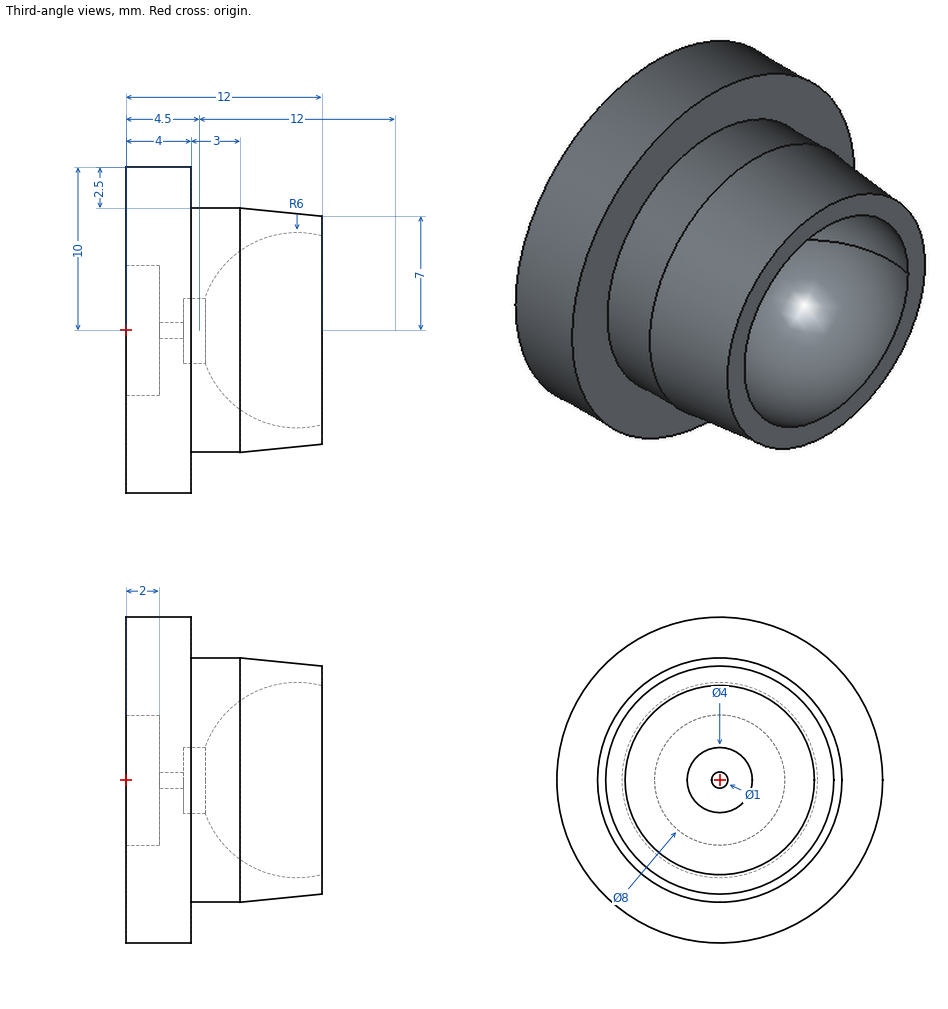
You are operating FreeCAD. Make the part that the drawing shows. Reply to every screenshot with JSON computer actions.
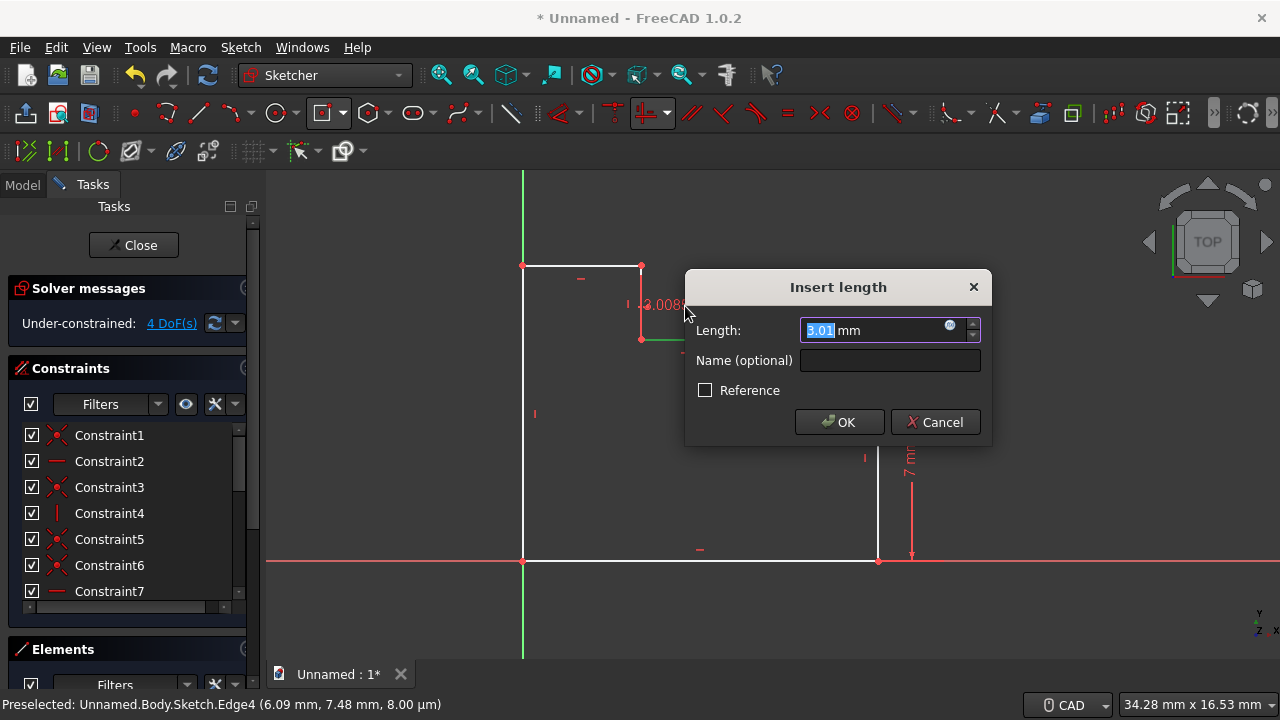
{"action": "type", "text": "3"}
{"action": "key", "text": "Return"}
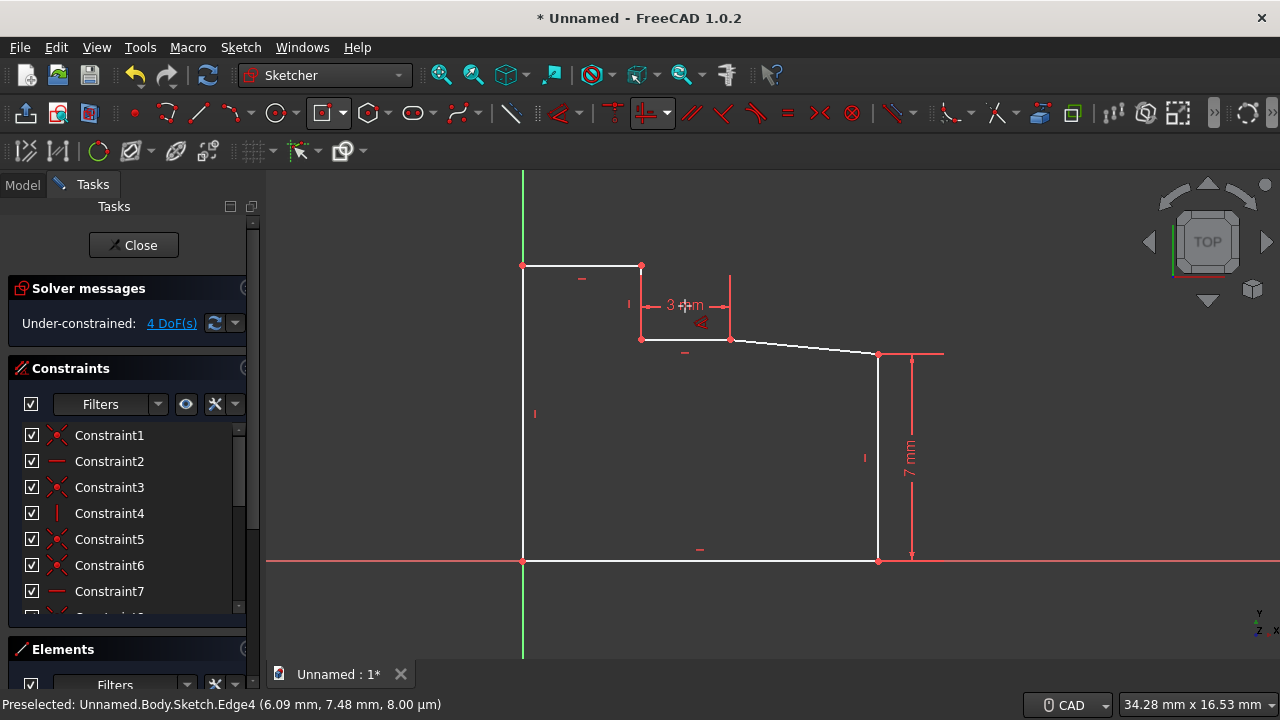
{"action": "left_click", "coordinate": [606, 266]}
{"action": "left_click", "coordinate": [582, 232]}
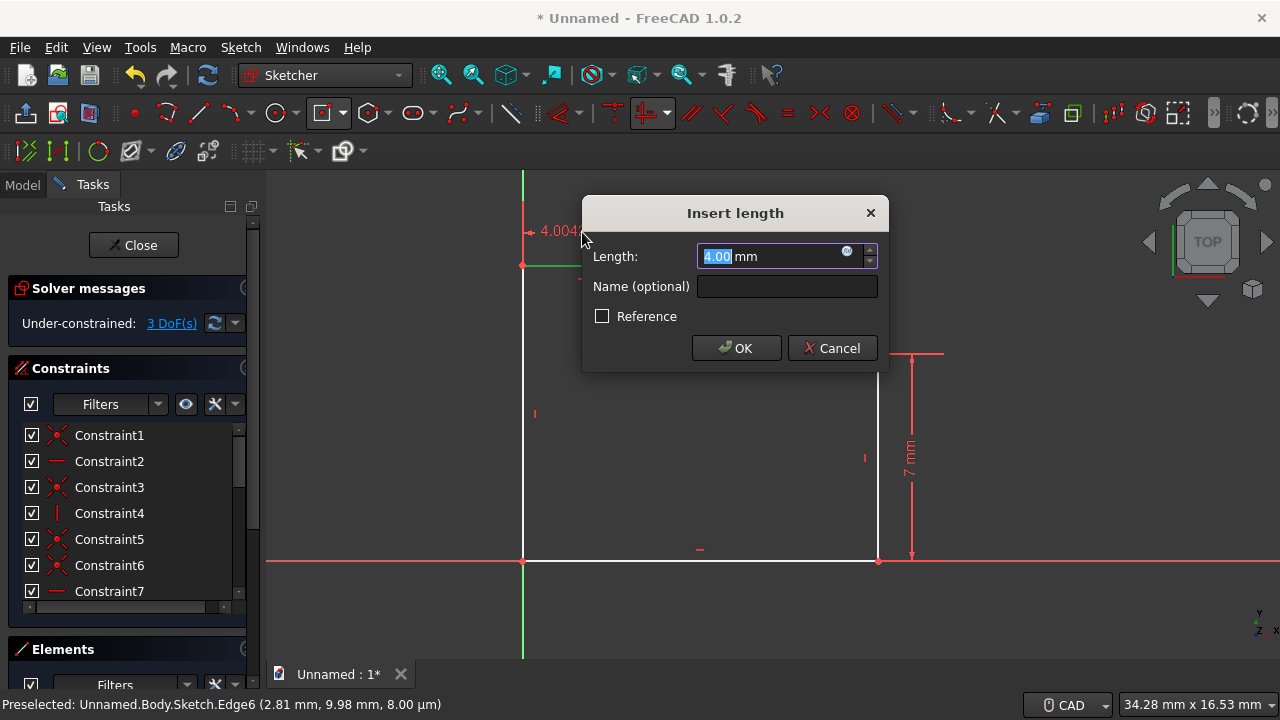
{"action": "type", "text": "4"}
{"action": "key", "text": "Return"}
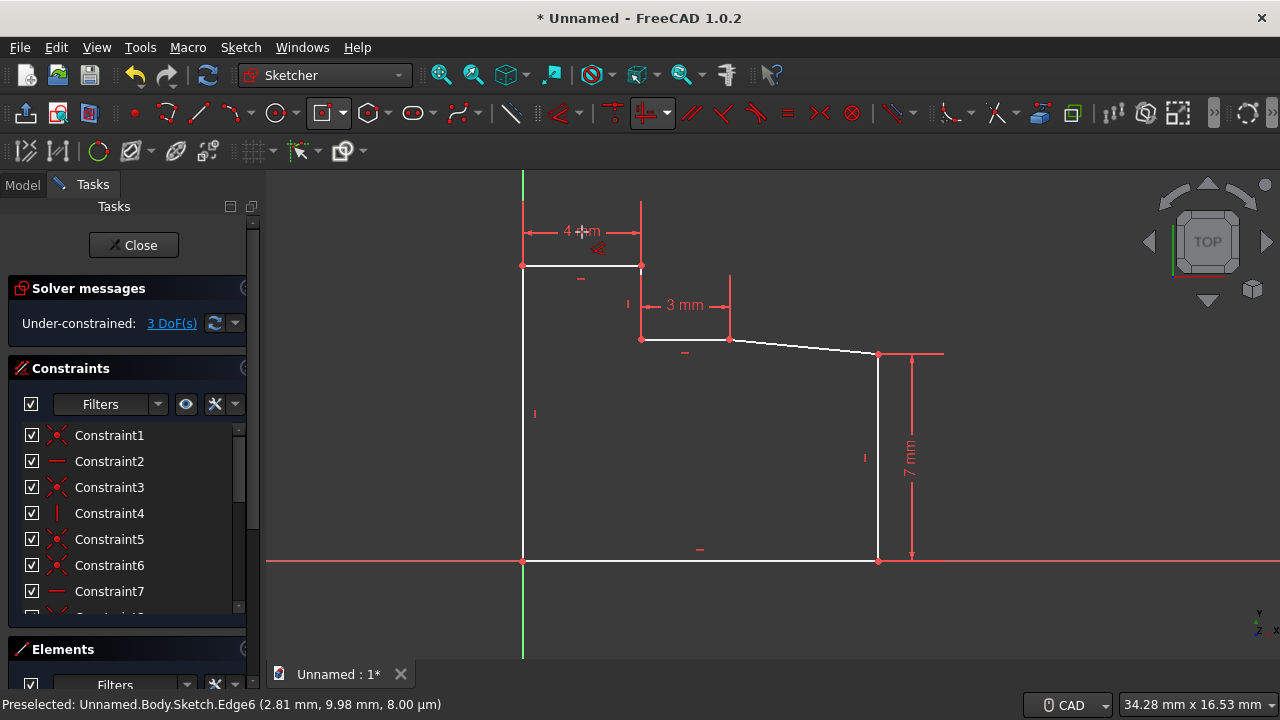
{"action": "left_click", "coordinate": [629, 561]}
{"action": "left_click", "coordinate": [700, 595]}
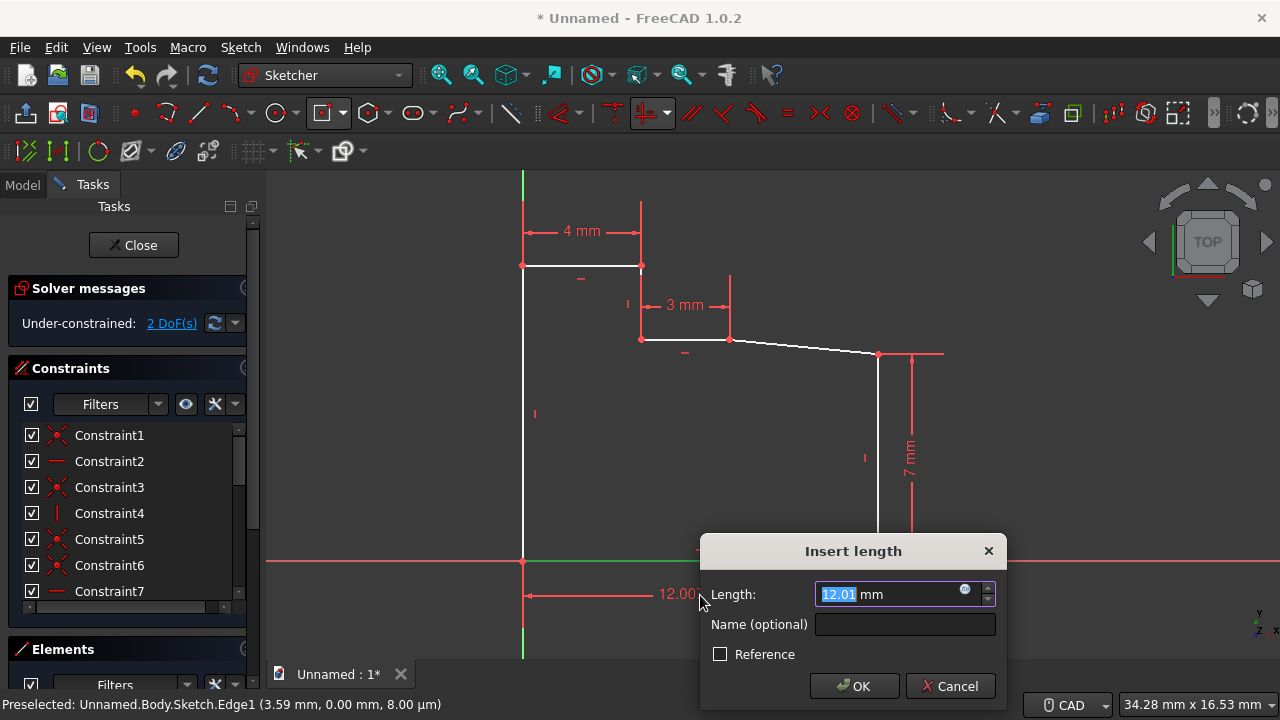
{"action": "type", "text": "12"}
{"action": "key", "text": "Return"}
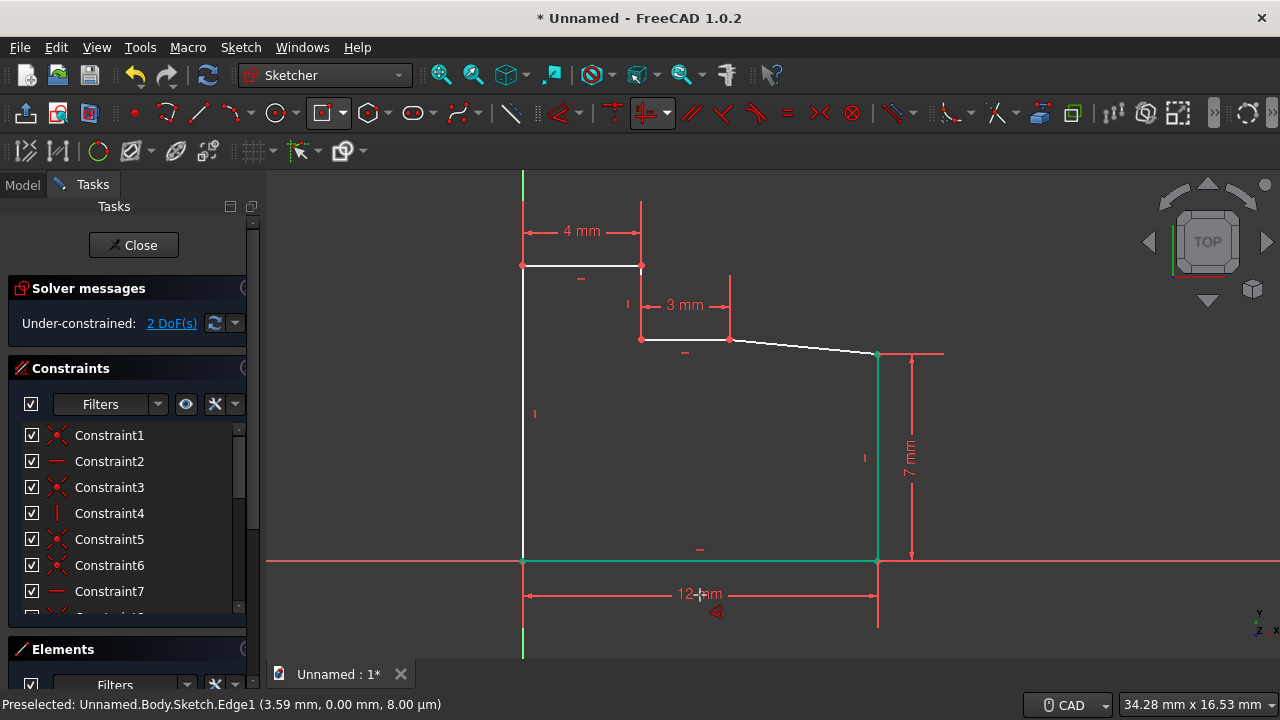
{"action": "left_click", "coordinate": [523, 355]}
{"action": "left_click", "coordinate": [489, 414]}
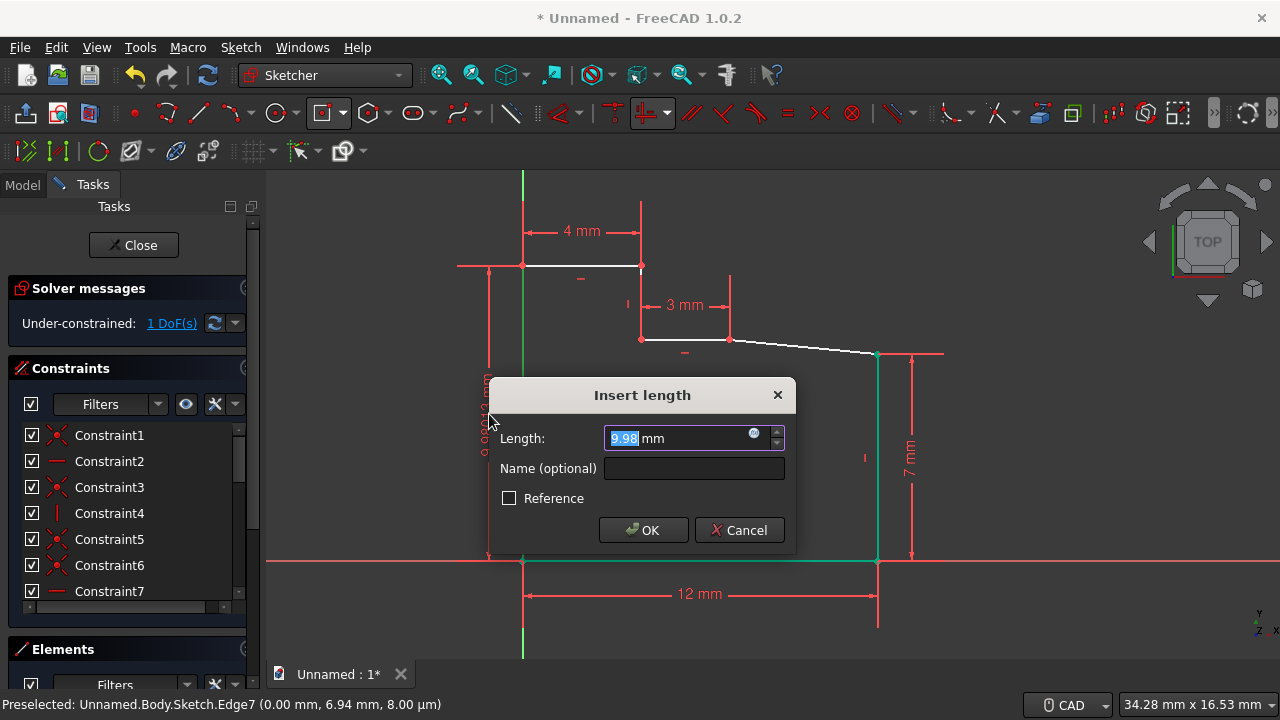
{"action": "type", "text": "10"}
{"action": "key", "text": "Return"}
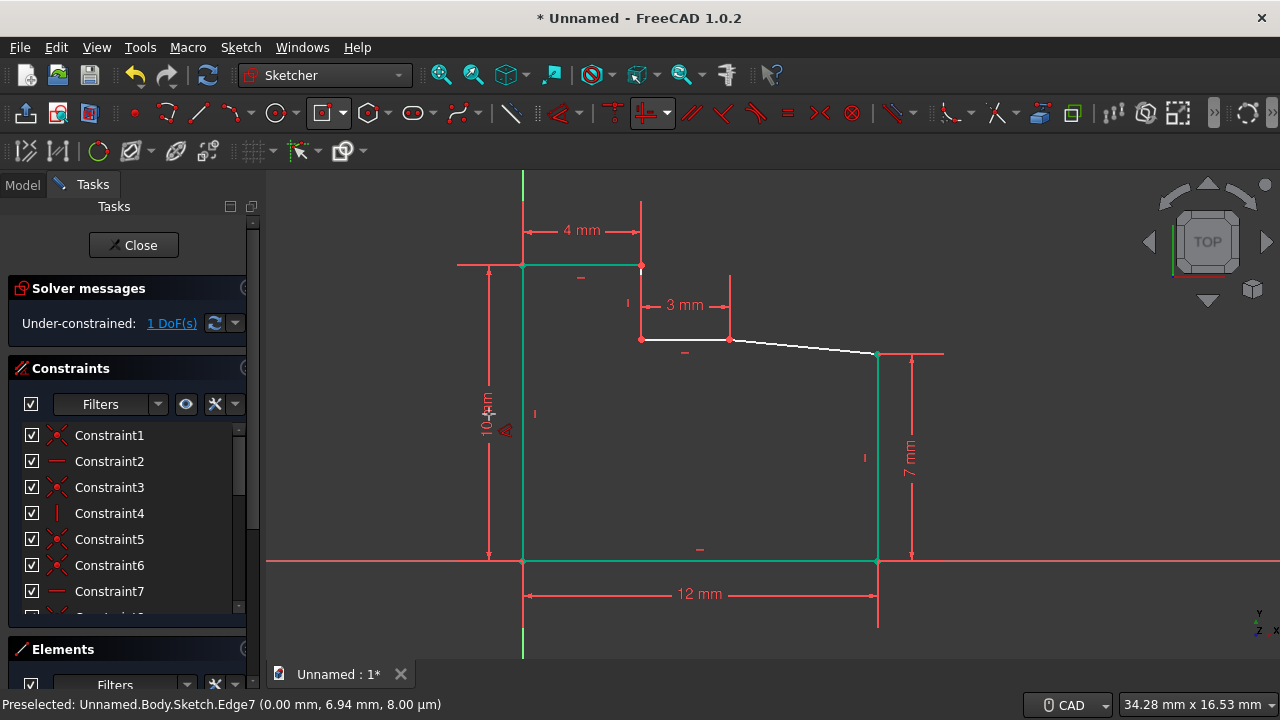
{"action": "left_click", "coordinate": [641, 318]}
{"action": "left_click", "coordinate": [607, 303]}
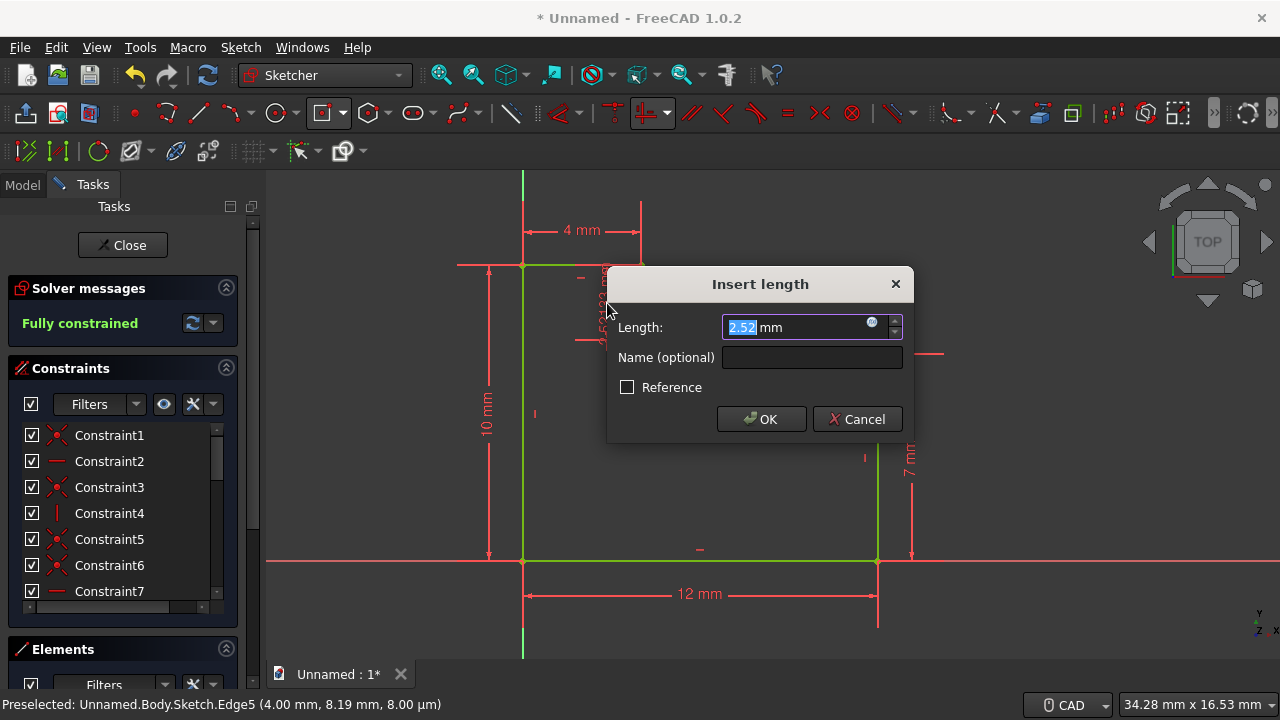
{"action": "type", "text": "2.5"}
{"action": "key", "text": "Return"}
{"action": "key", "text": "Escape"}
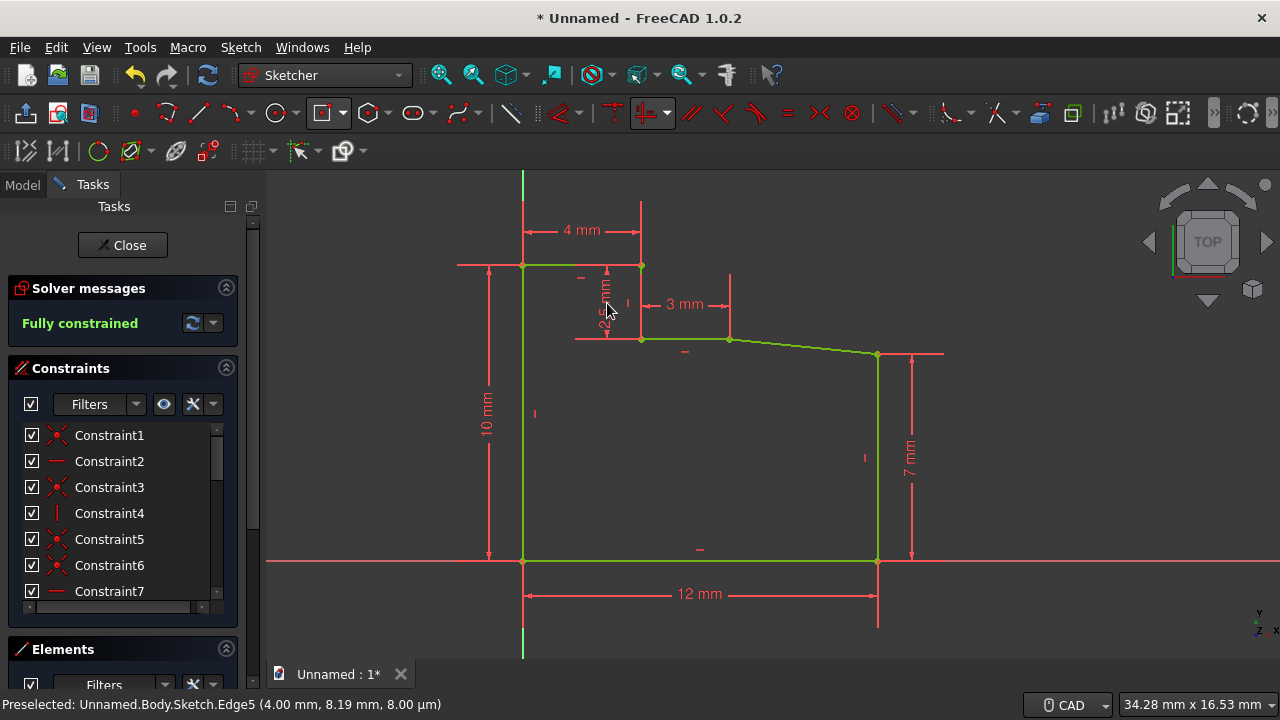
{"action": "left_click", "coordinate": [123, 245]}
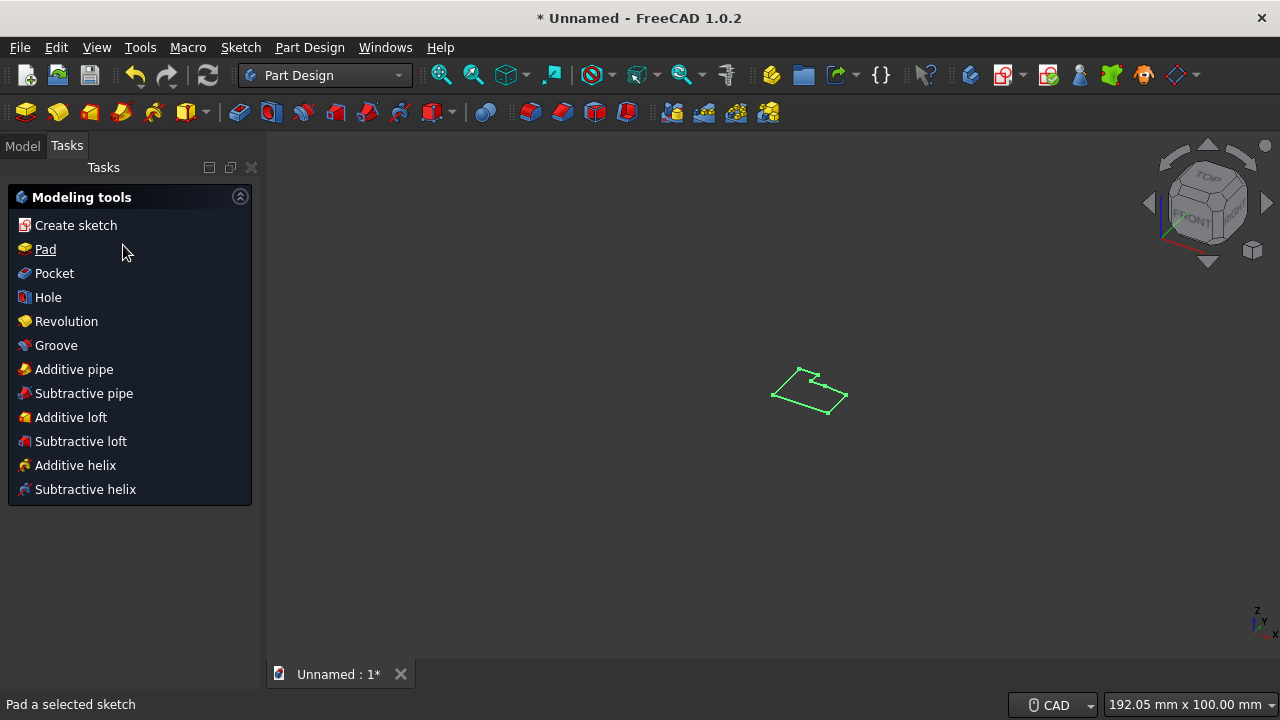
{"action": "left_click", "coordinate": [58, 112]}